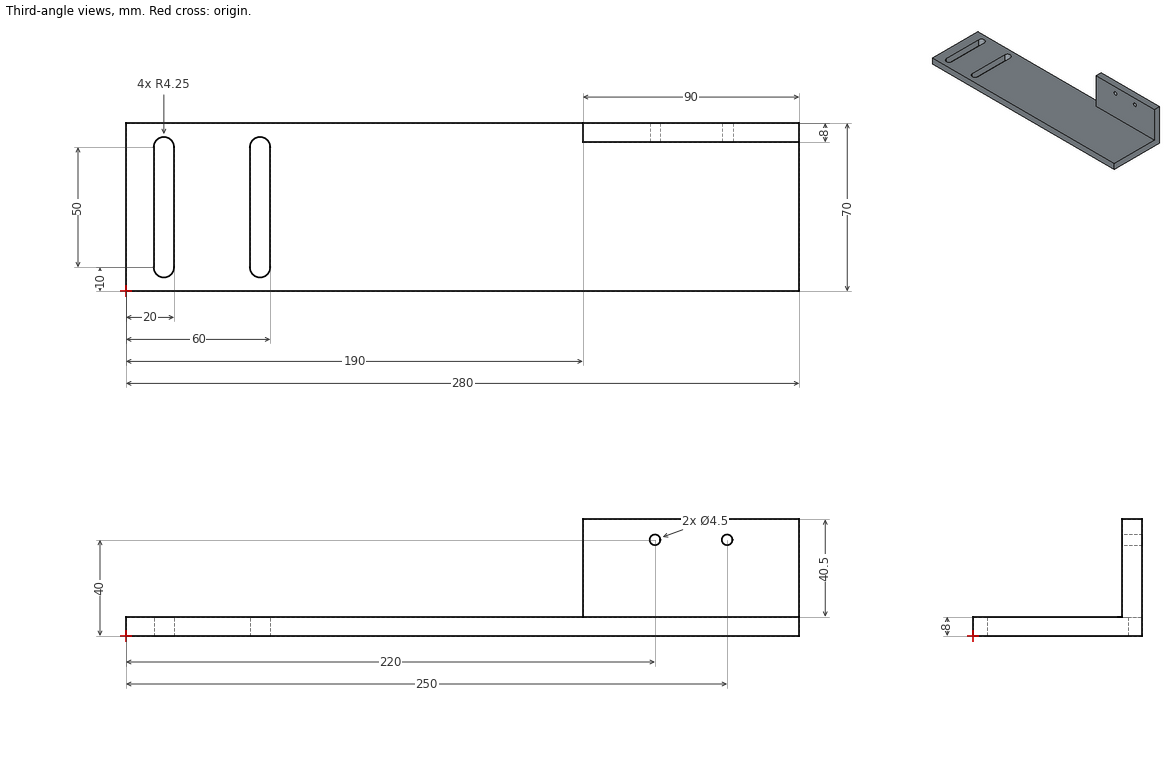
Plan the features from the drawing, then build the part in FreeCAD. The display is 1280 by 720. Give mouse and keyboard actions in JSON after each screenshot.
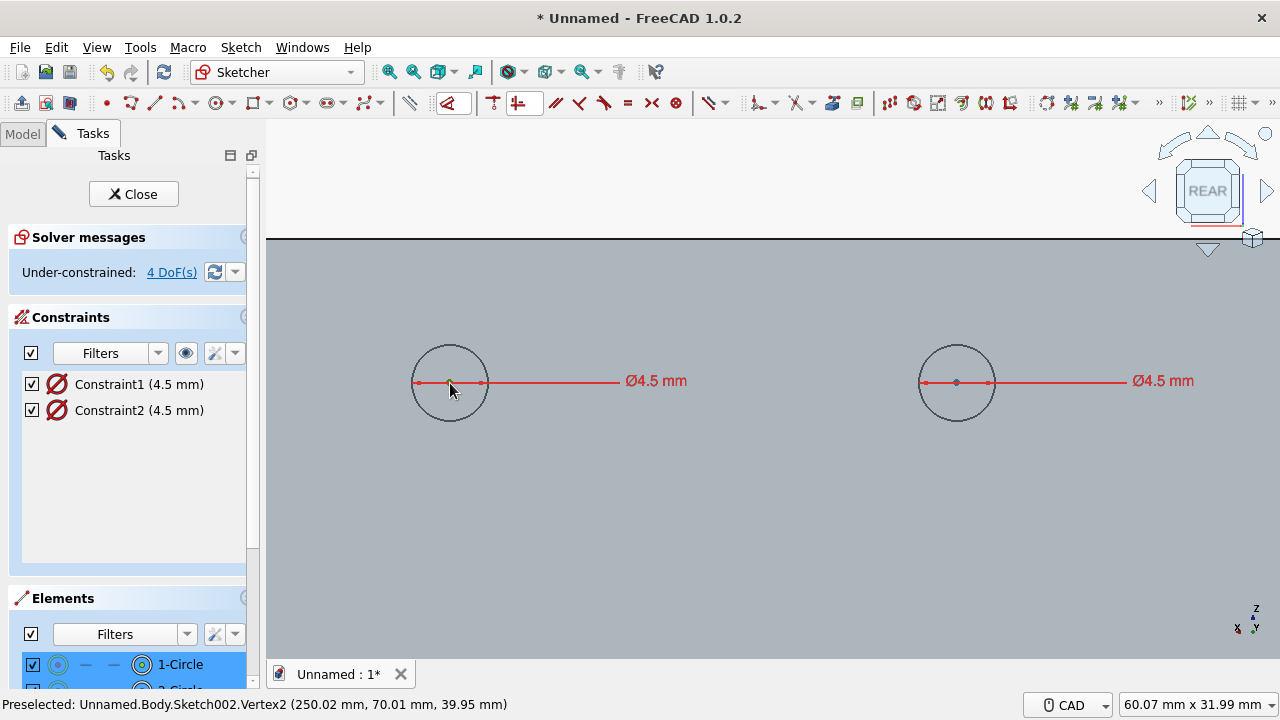
{"action": "key", "text": "h"}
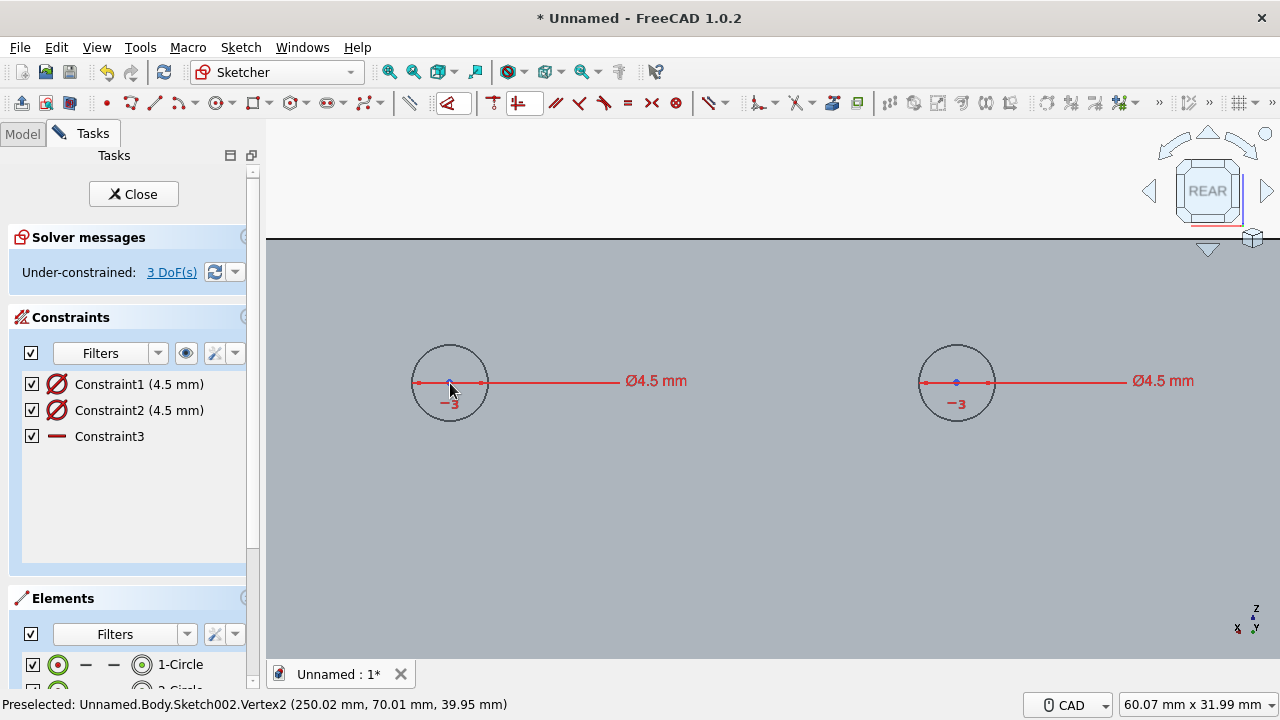
{"action": "left_click", "coordinate": [957, 383]}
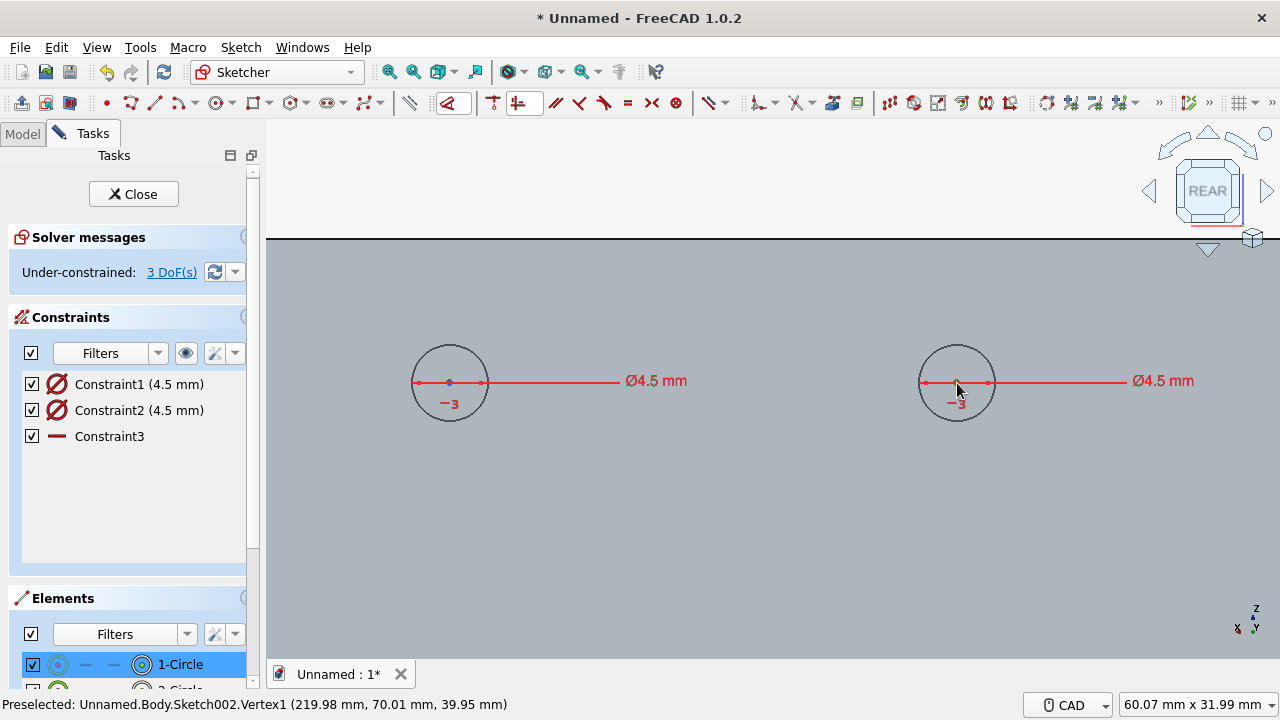
{"action": "key", "text": "i"}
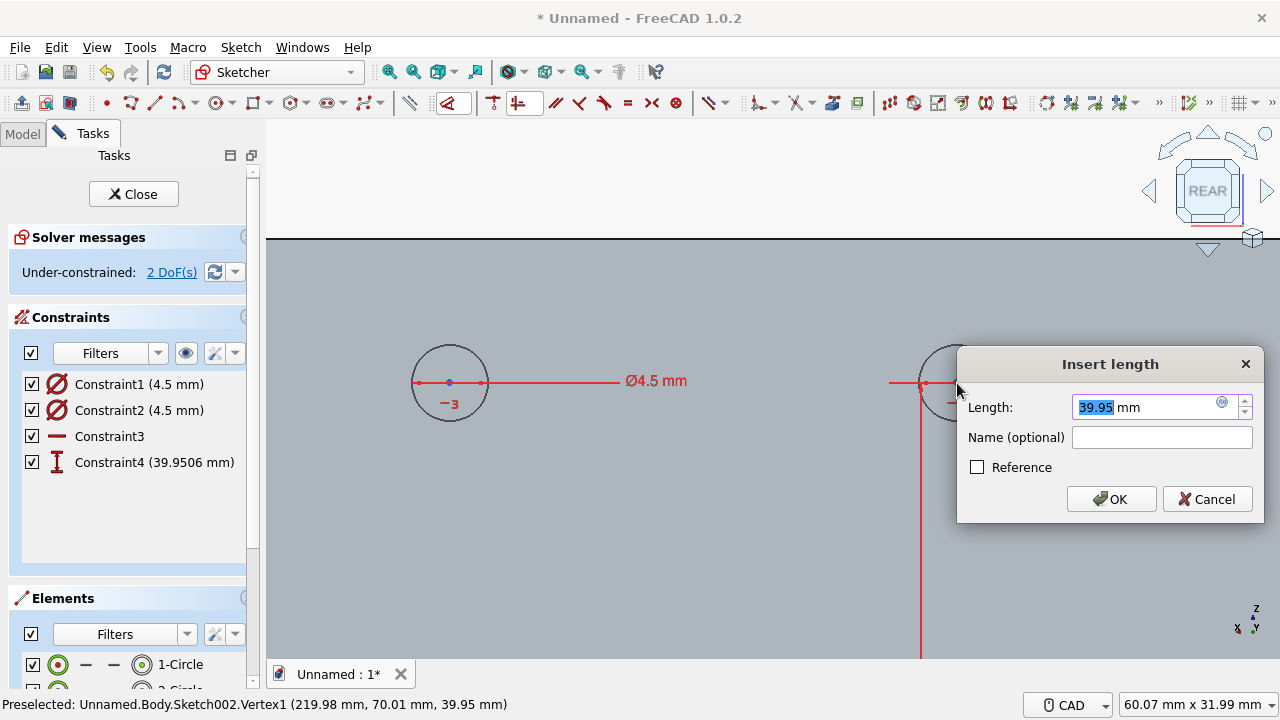
{"action": "type", "text": "40"}
{"action": "key", "text": "Return"}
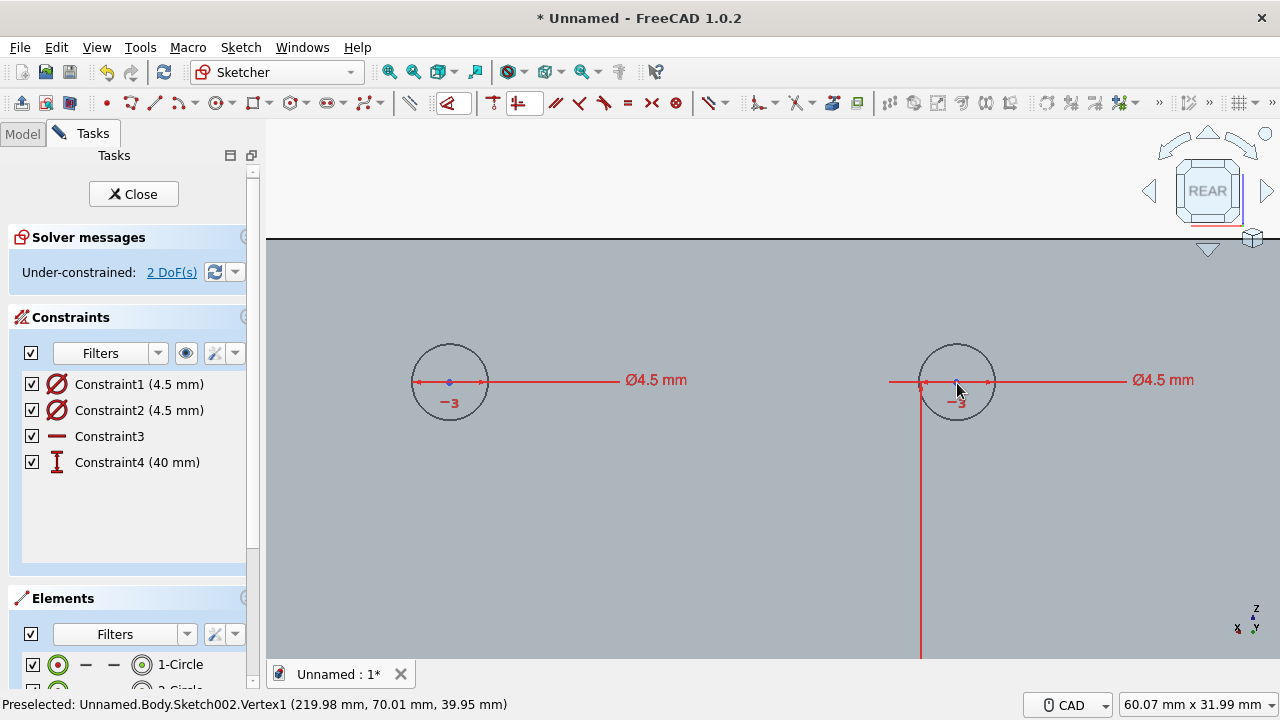
{"action": "left_click", "coordinate": [957, 382]}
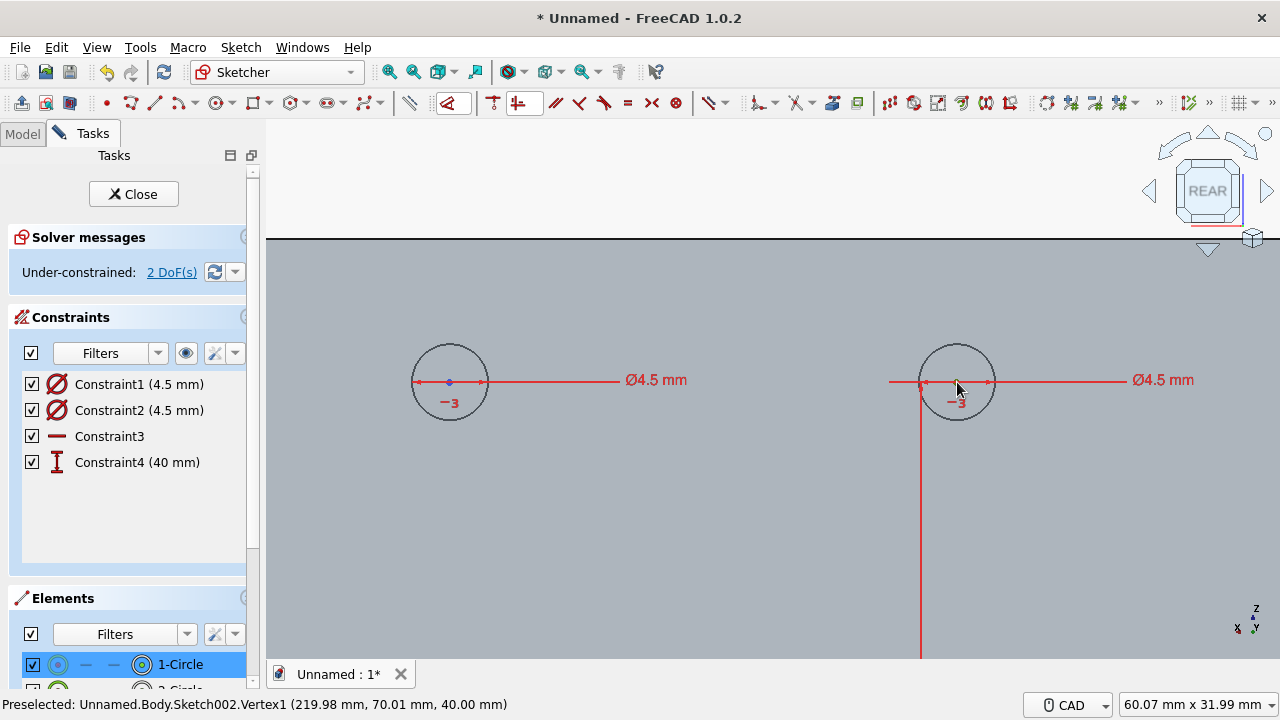
{"action": "key", "text": "l"}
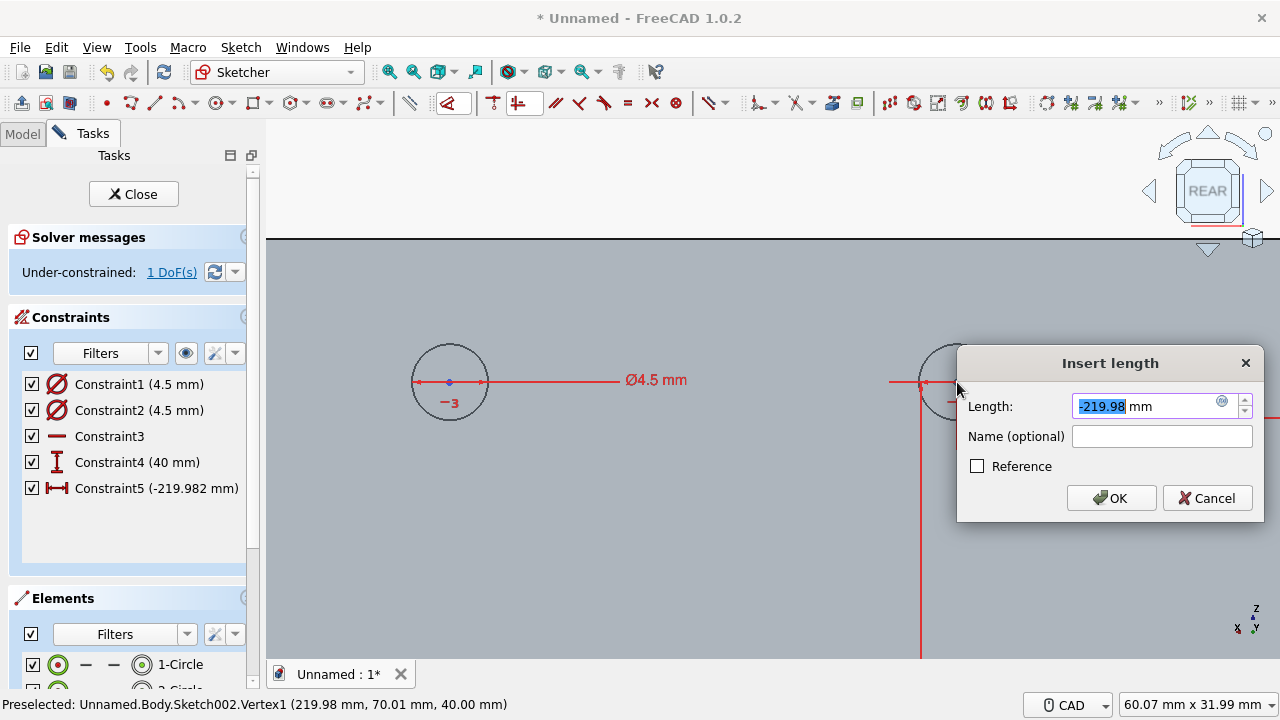
{"action": "type", "text": "-220"}
{"action": "key", "text": "Return"}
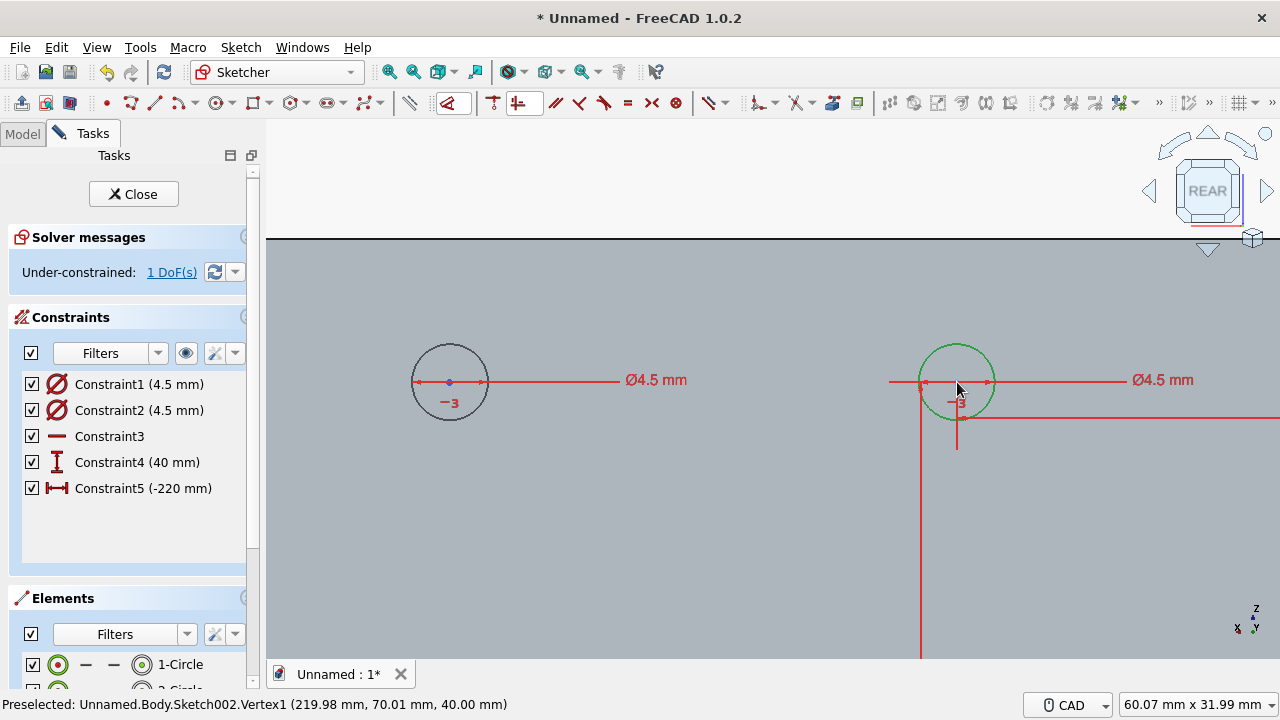
{"action": "left_click", "coordinate": [450, 382]}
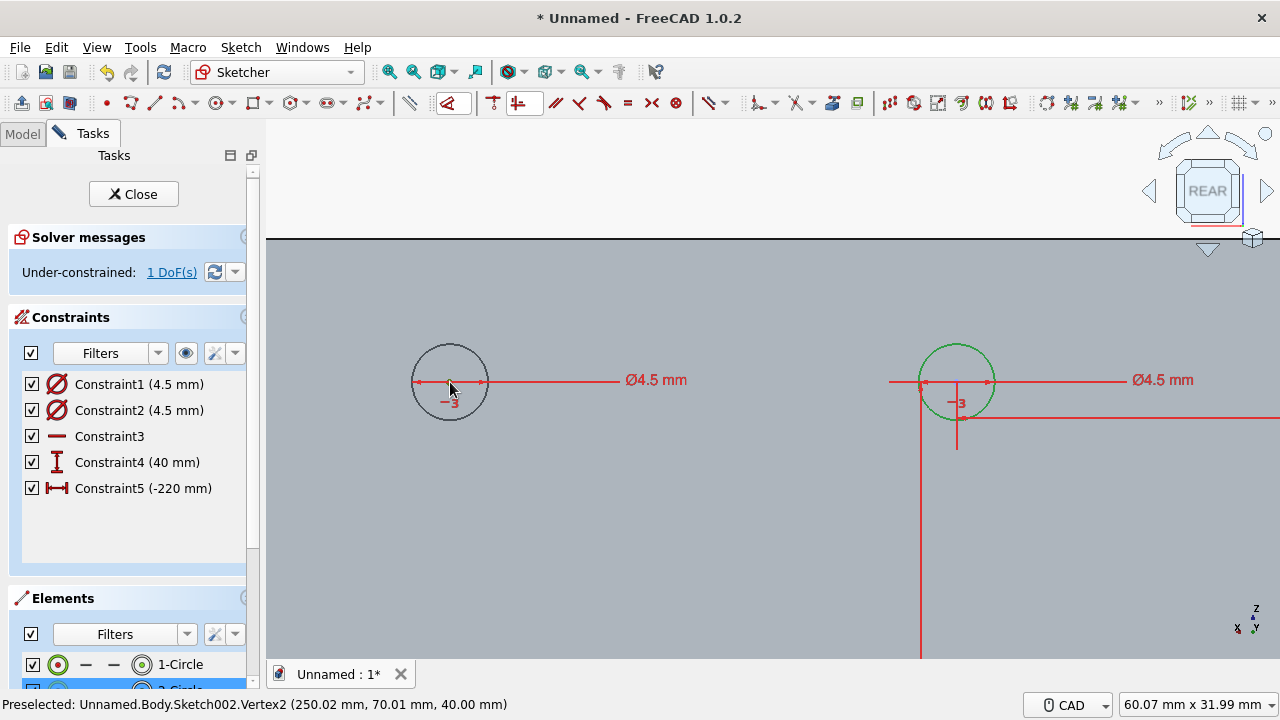
{"action": "key", "text": "l"}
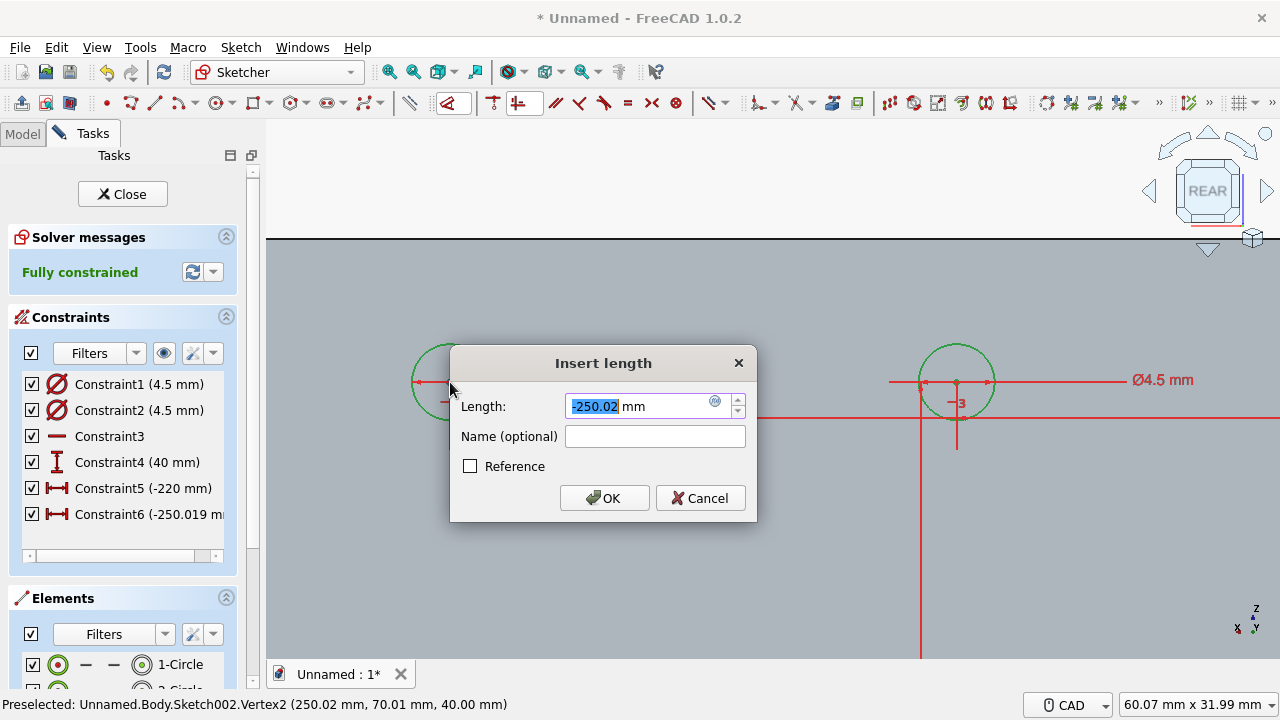
{"action": "type", "text": "-250"}
{"action": "key", "text": "Return"}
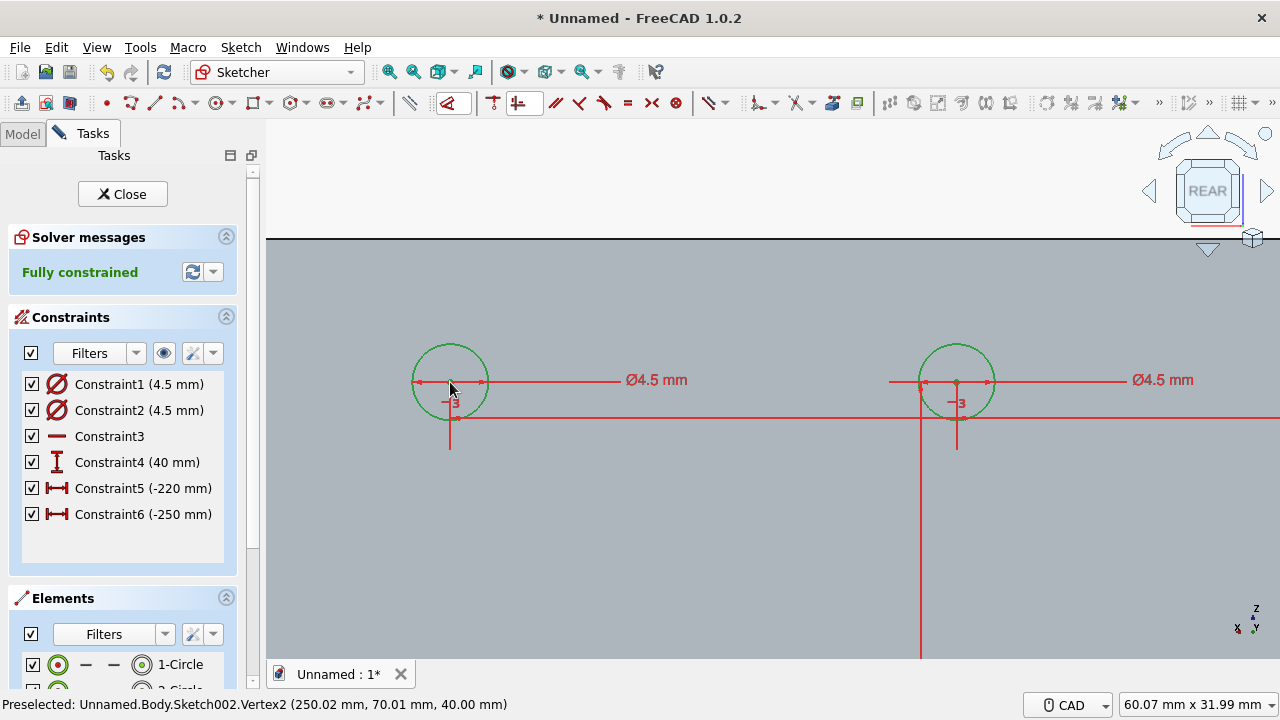
{"action": "left_click", "coordinate": [123, 194]}